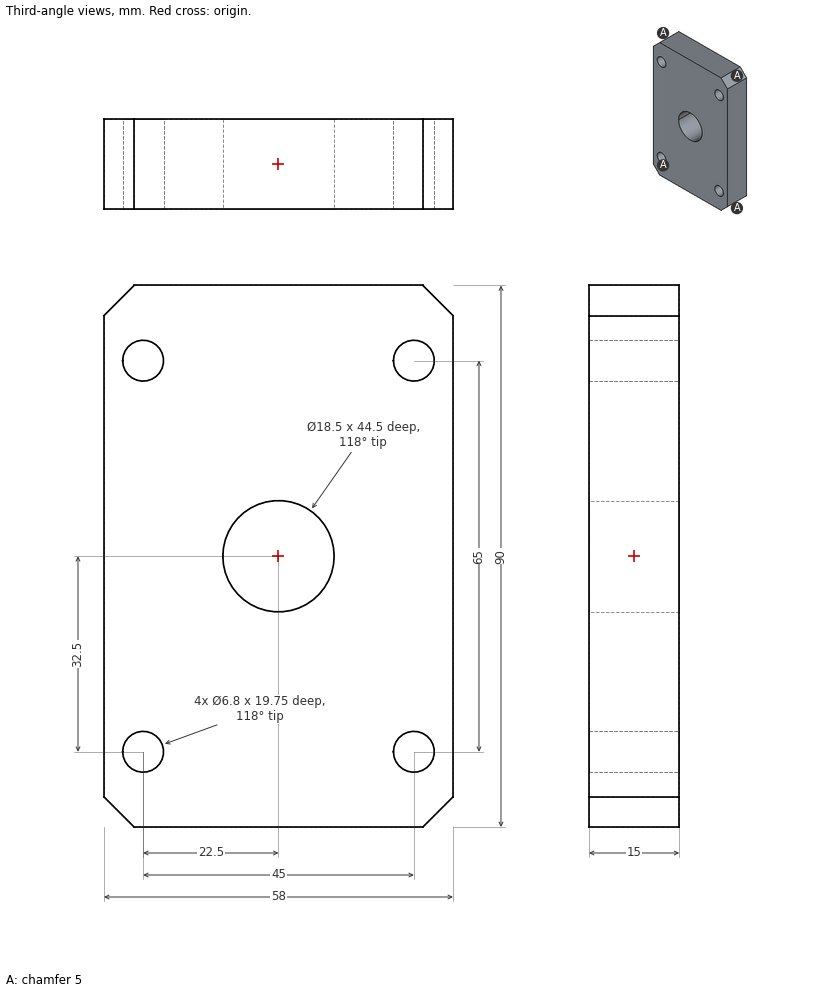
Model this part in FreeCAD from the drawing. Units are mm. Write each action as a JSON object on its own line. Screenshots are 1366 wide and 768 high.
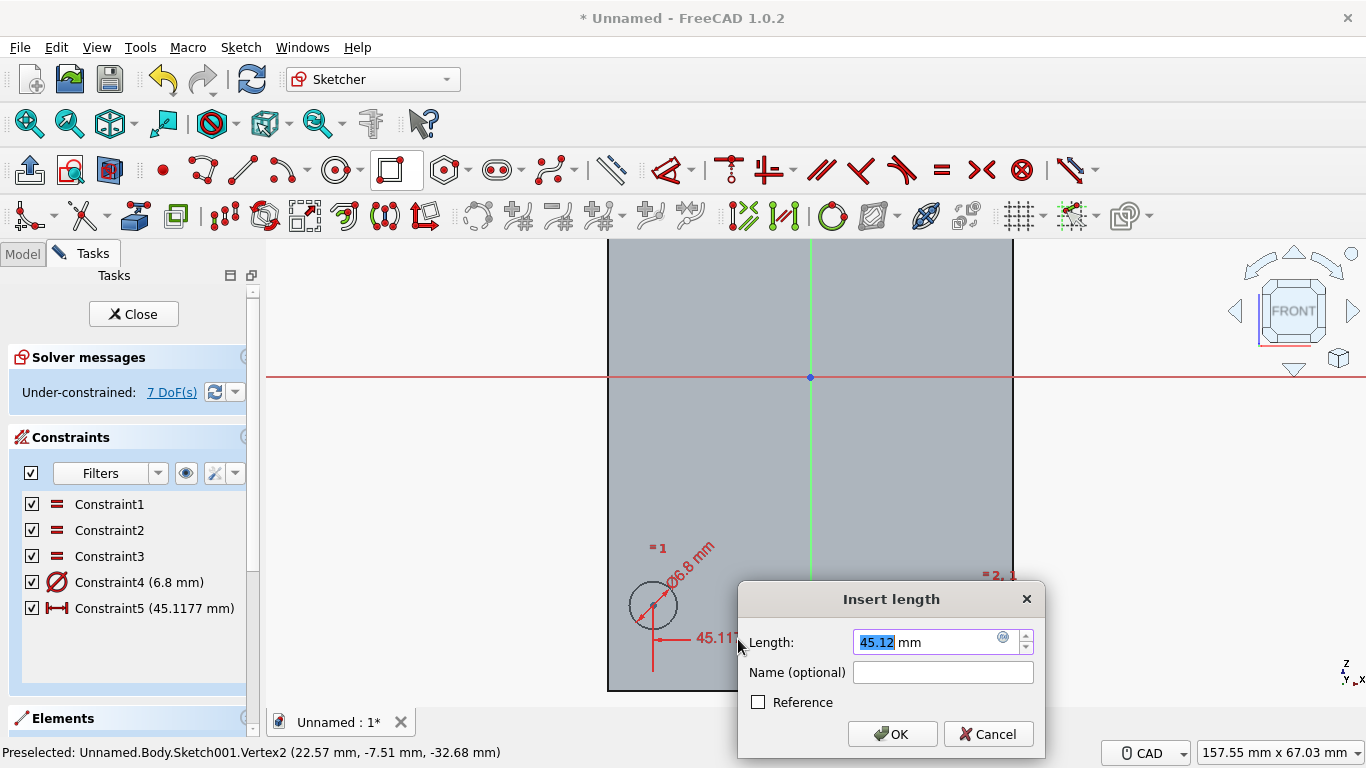
{"action": "type", "text": "45"}
{"action": "key", "text": "Return"}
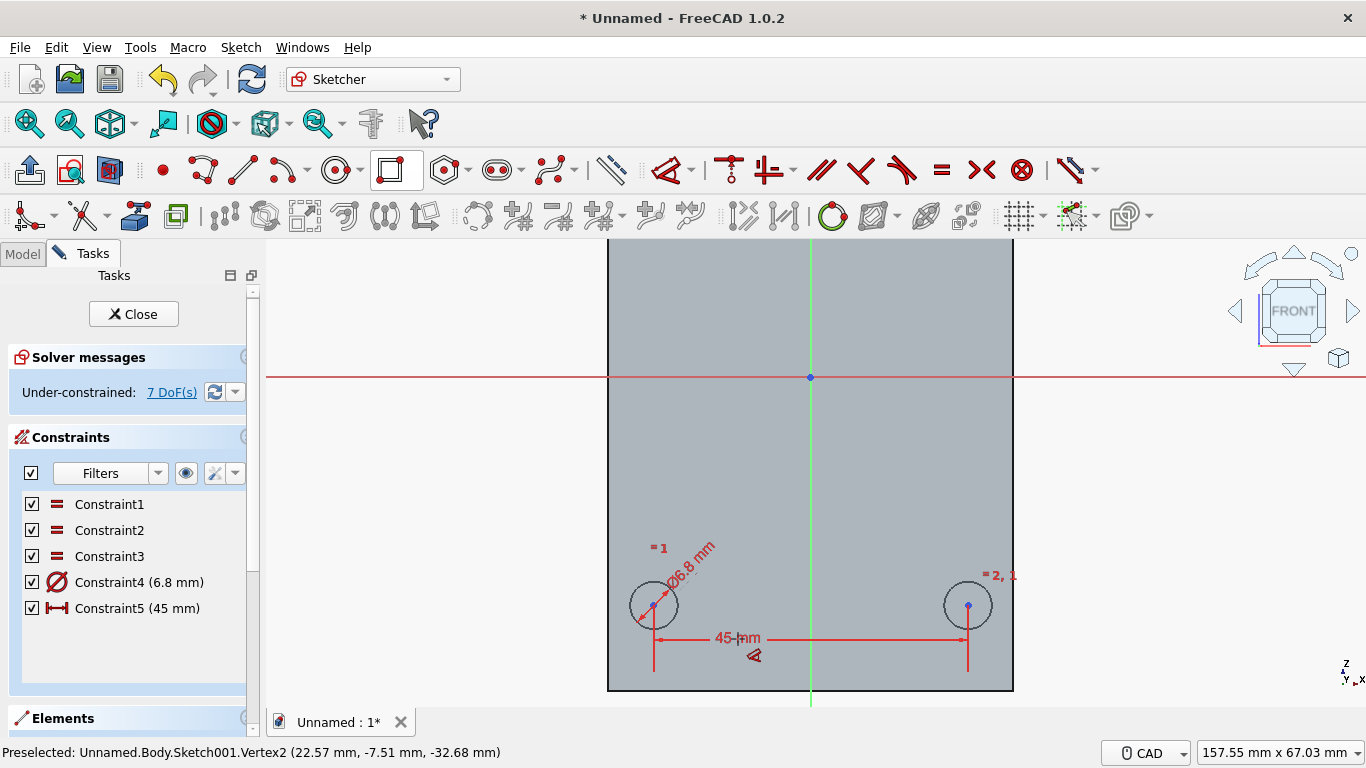
{"action": "left_click", "coordinate": [654, 605]}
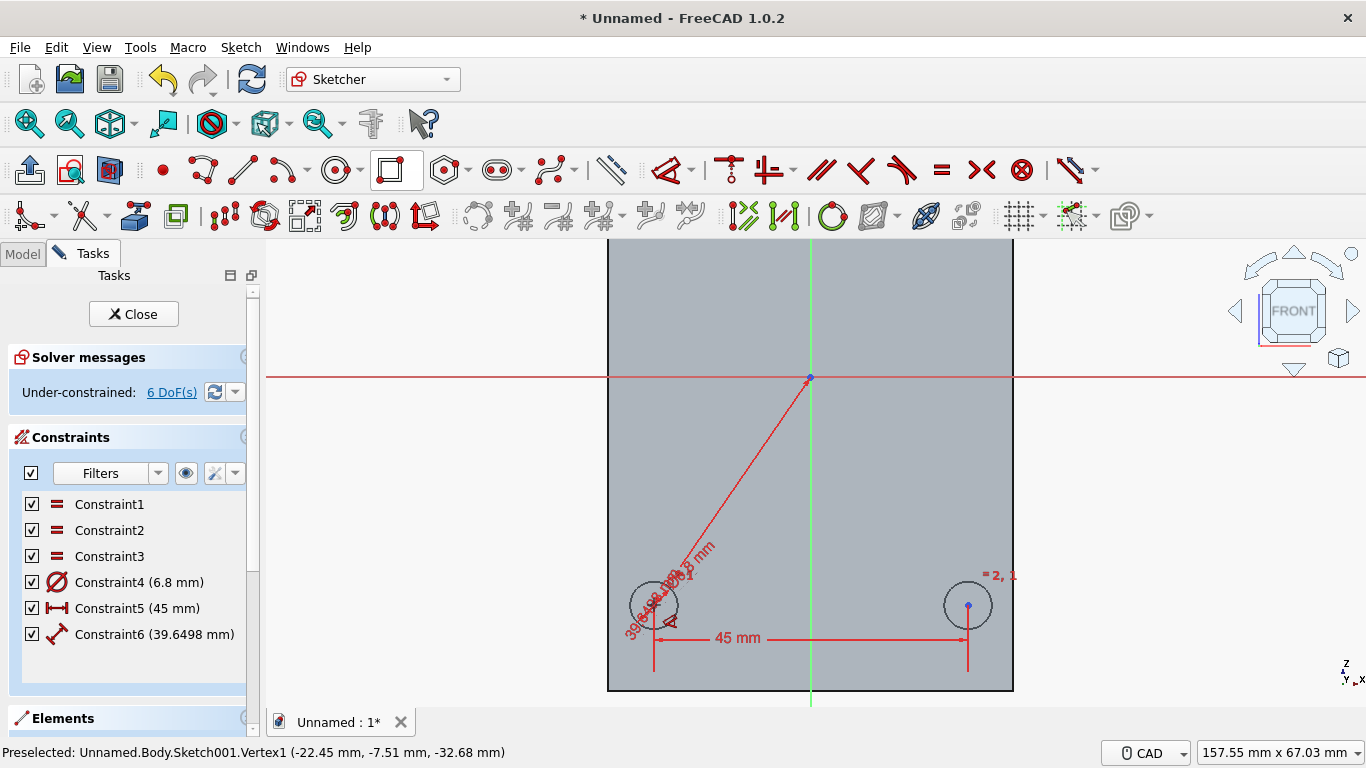
{"action": "scroll", "coordinate": [671, 589], "scroll_direction": "down", "scroll_amount": 3}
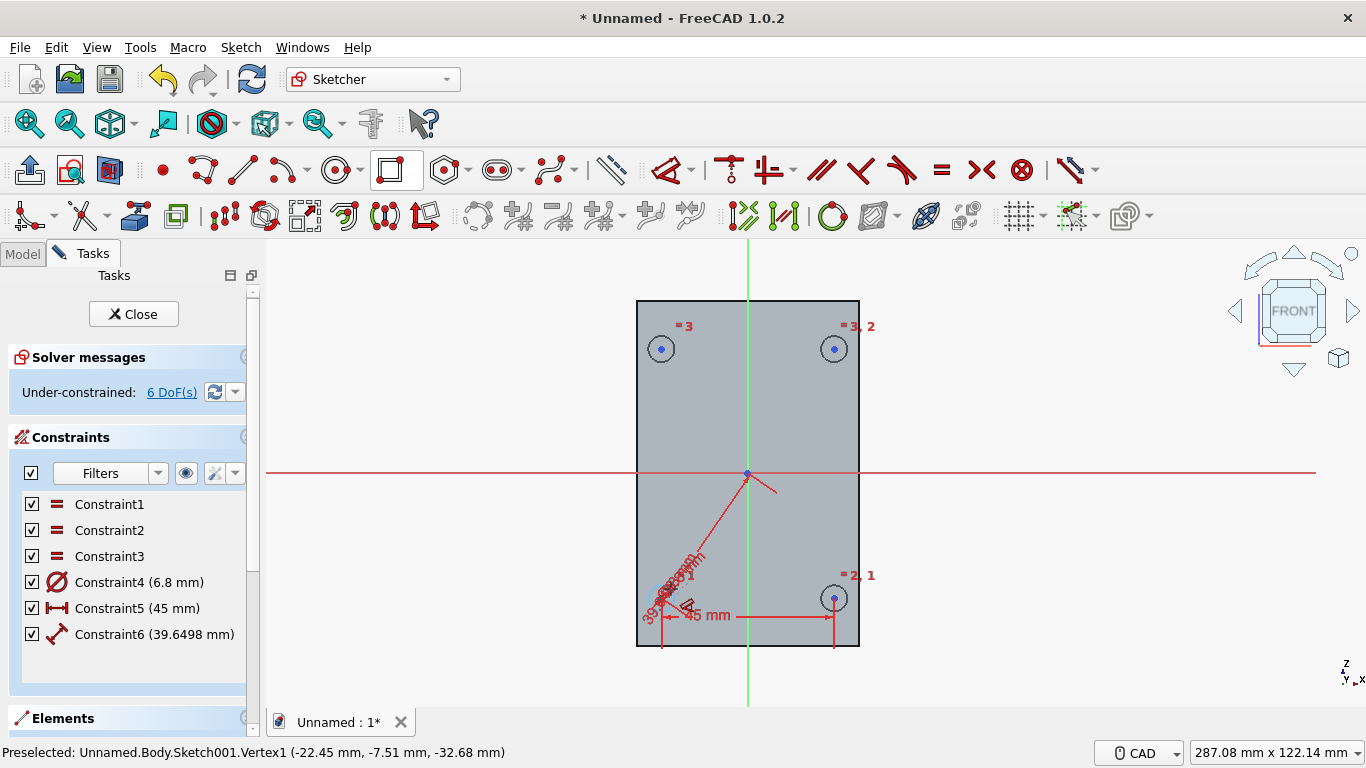
{"action": "left_click", "coordinate": [834, 349]}
{"action": "left_click", "coordinate": [788, 632]}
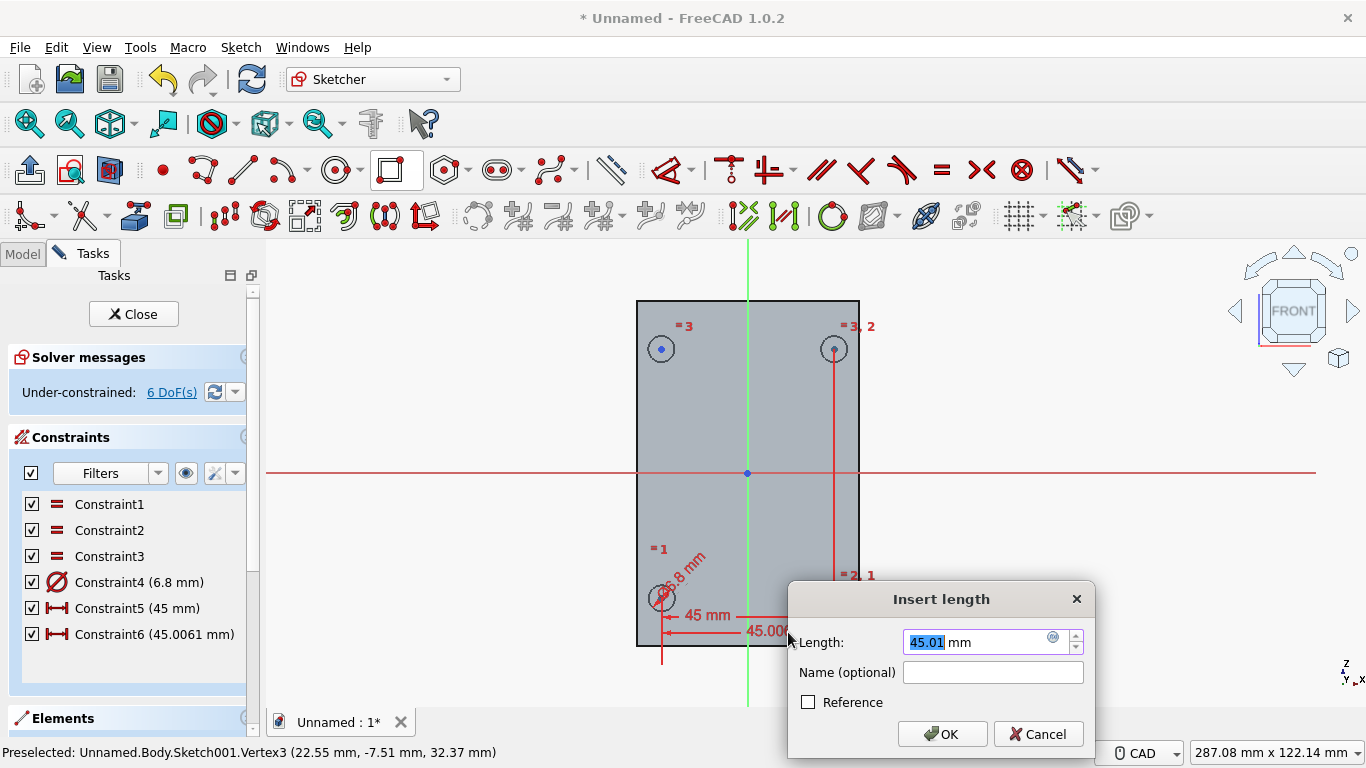
{"action": "type", "text": "45"}
{"action": "key", "text": "Return"}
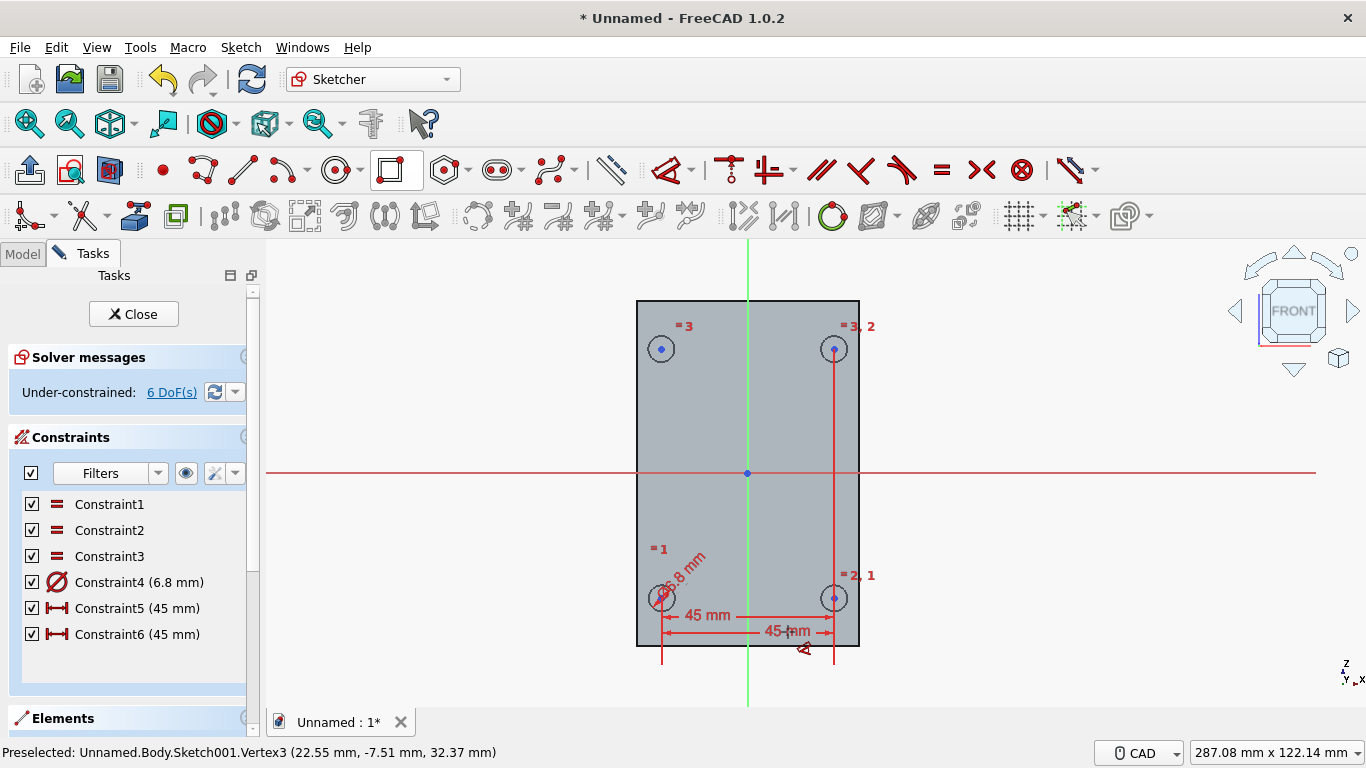
{"action": "left_click", "coordinate": [834, 598]}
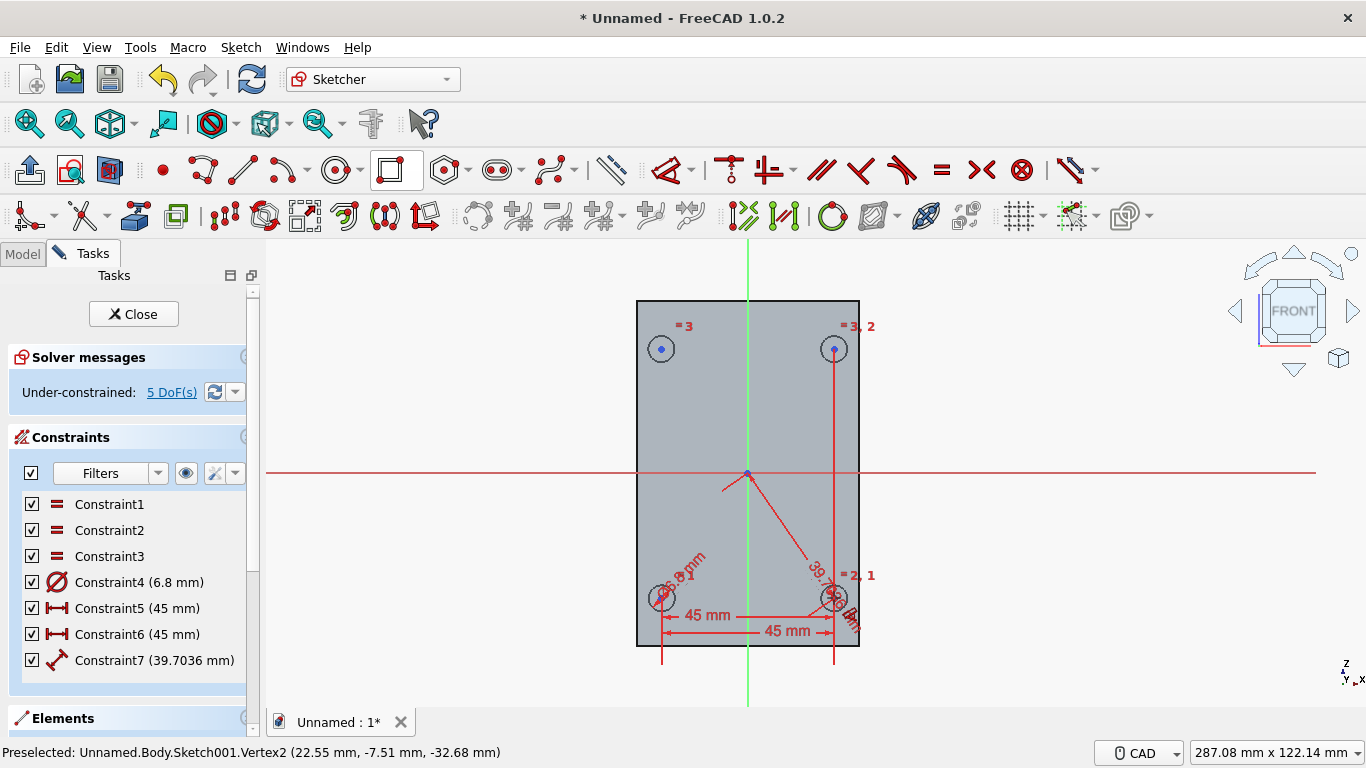
{"action": "left_click", "coordinate": [834, 349]}
{"action": "left_click", "coordinate": [868, 416]}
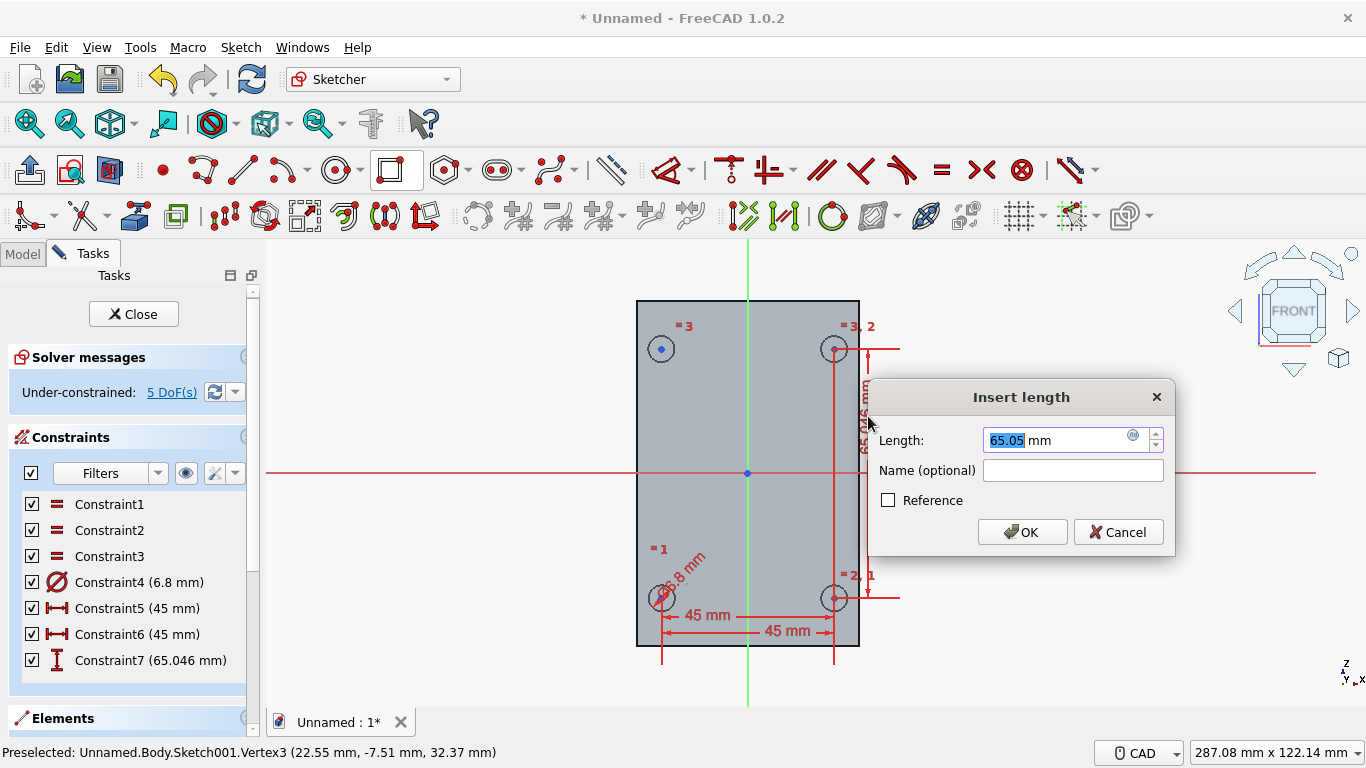
{"action": "type", "text": "65"}
{"action": "key", "text": "Return"}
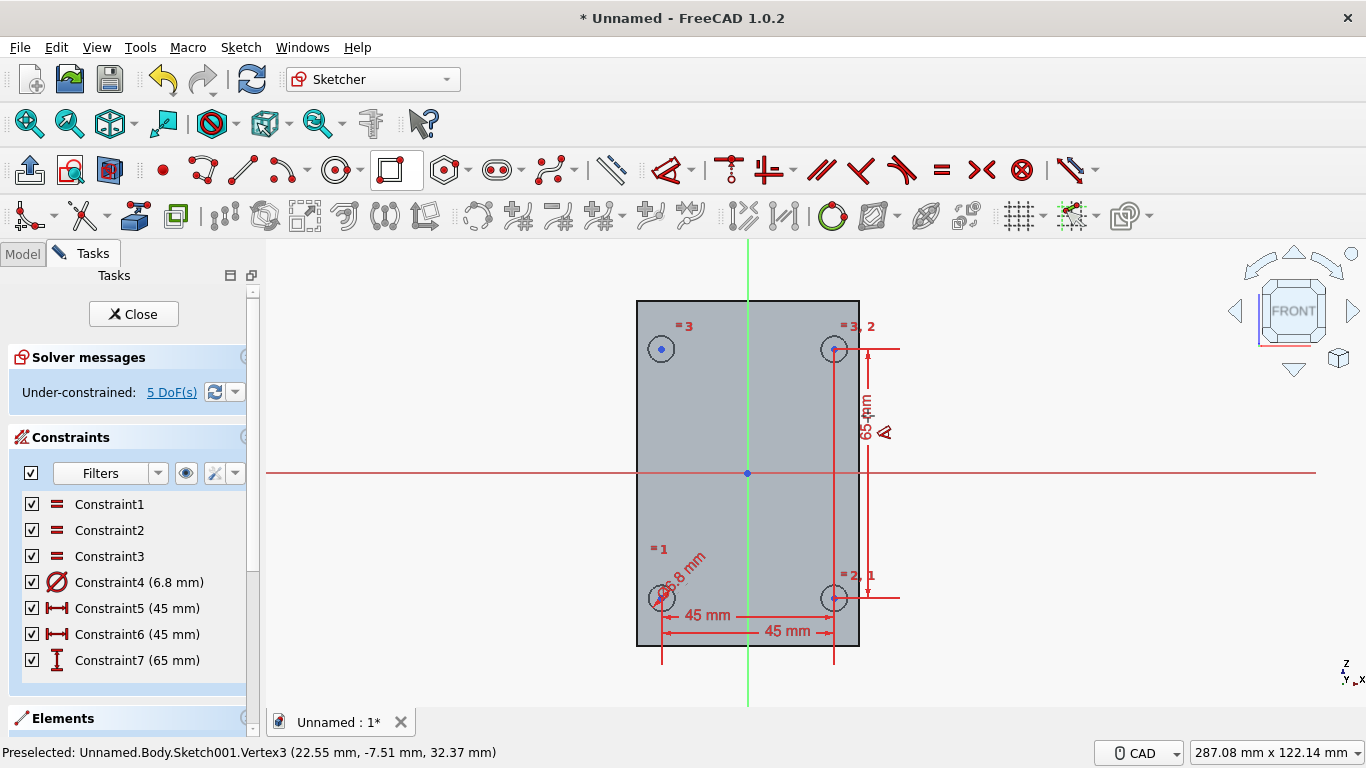
{"action": "left_click", "coordinate": [662, 598]}